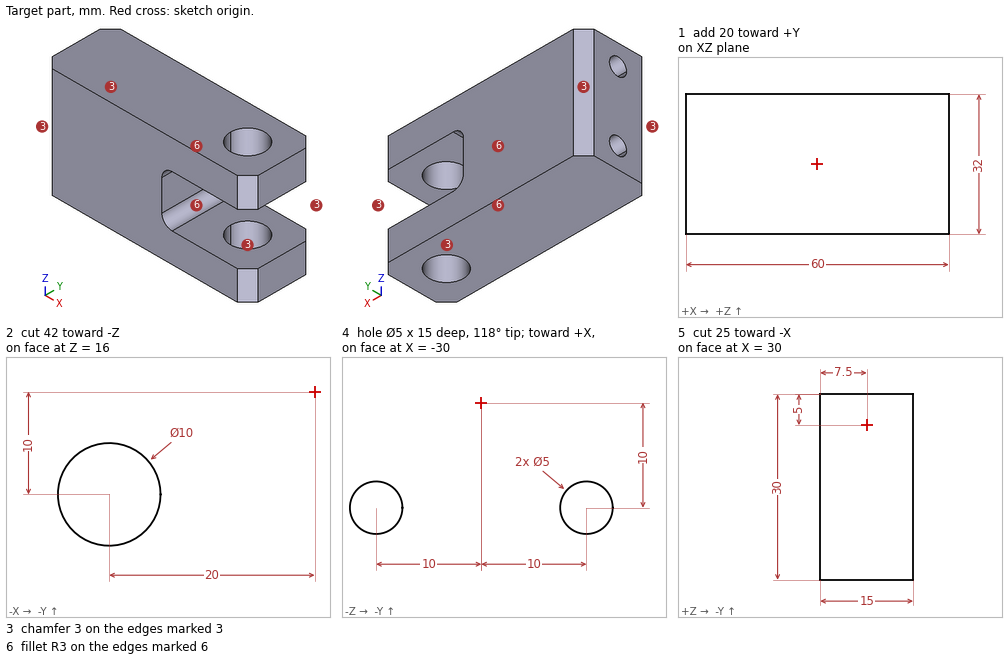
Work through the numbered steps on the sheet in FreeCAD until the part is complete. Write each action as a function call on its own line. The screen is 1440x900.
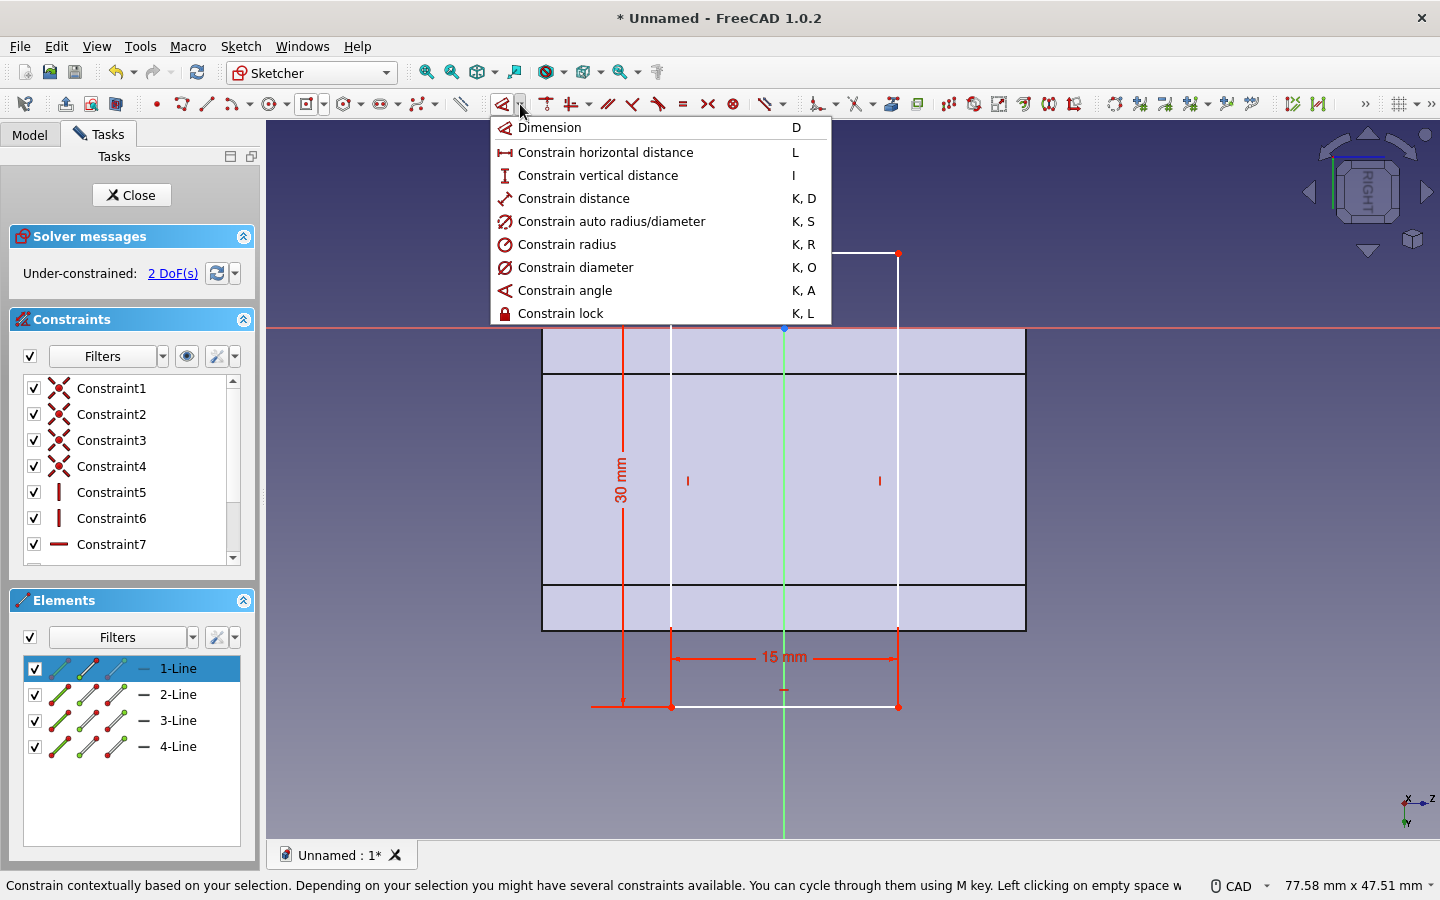
click(661, 176)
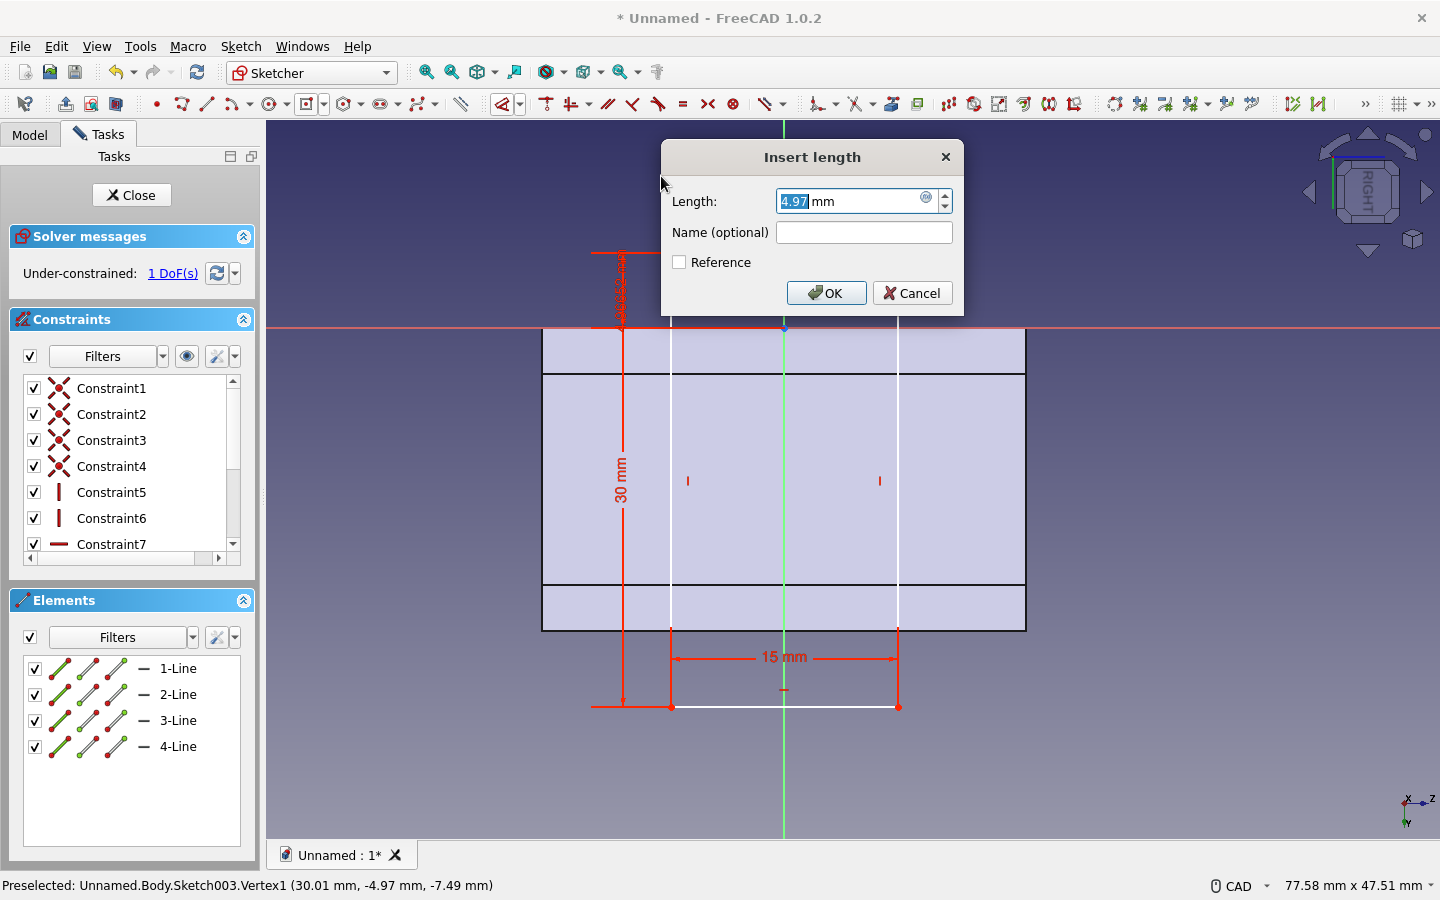
text(5)
key(Return)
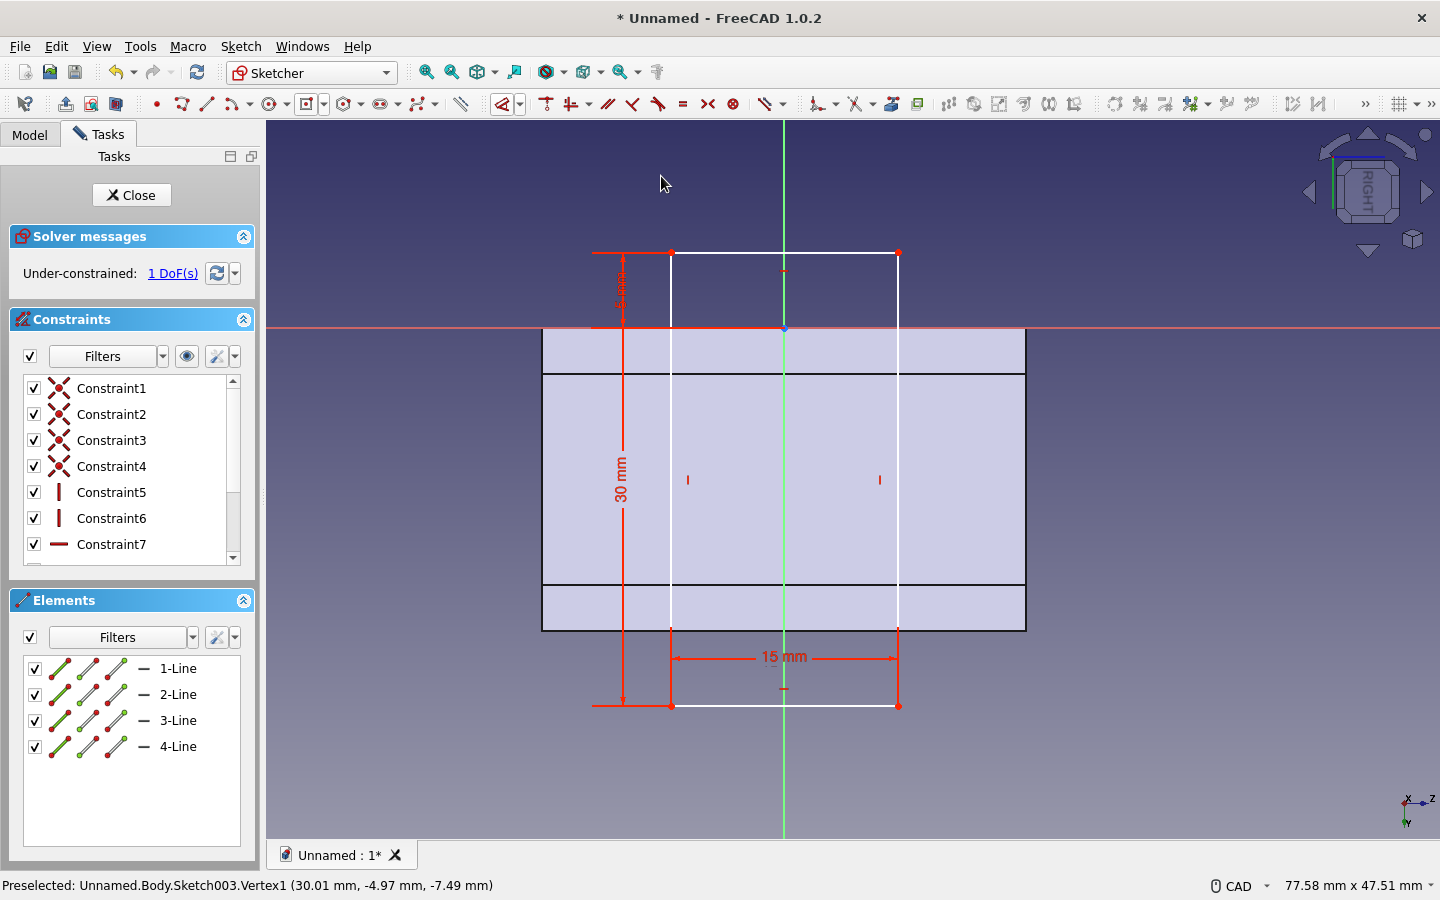
click(671, 253)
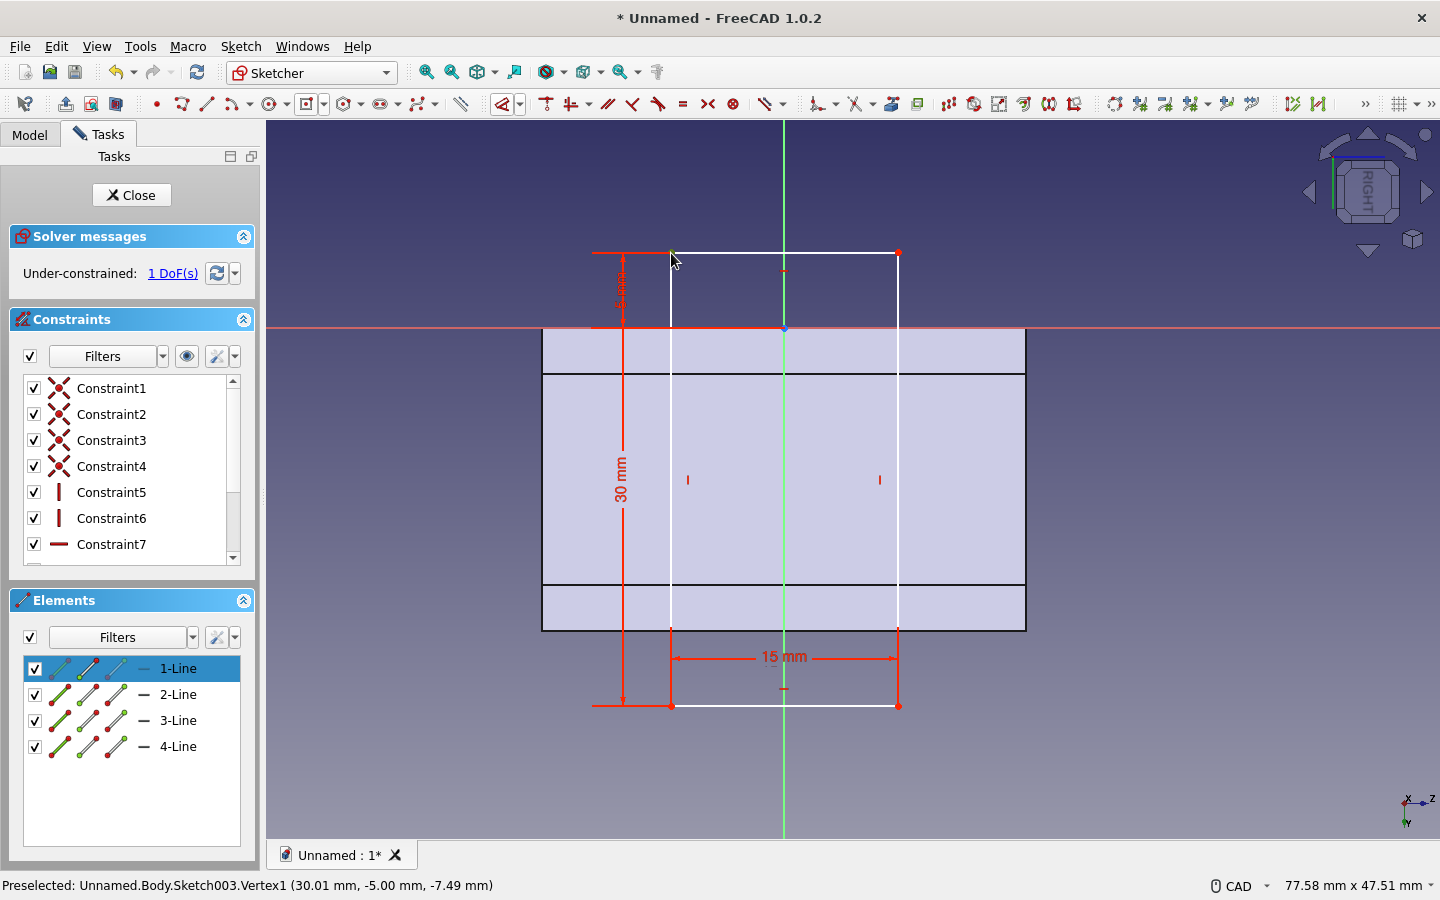
click(520, 104)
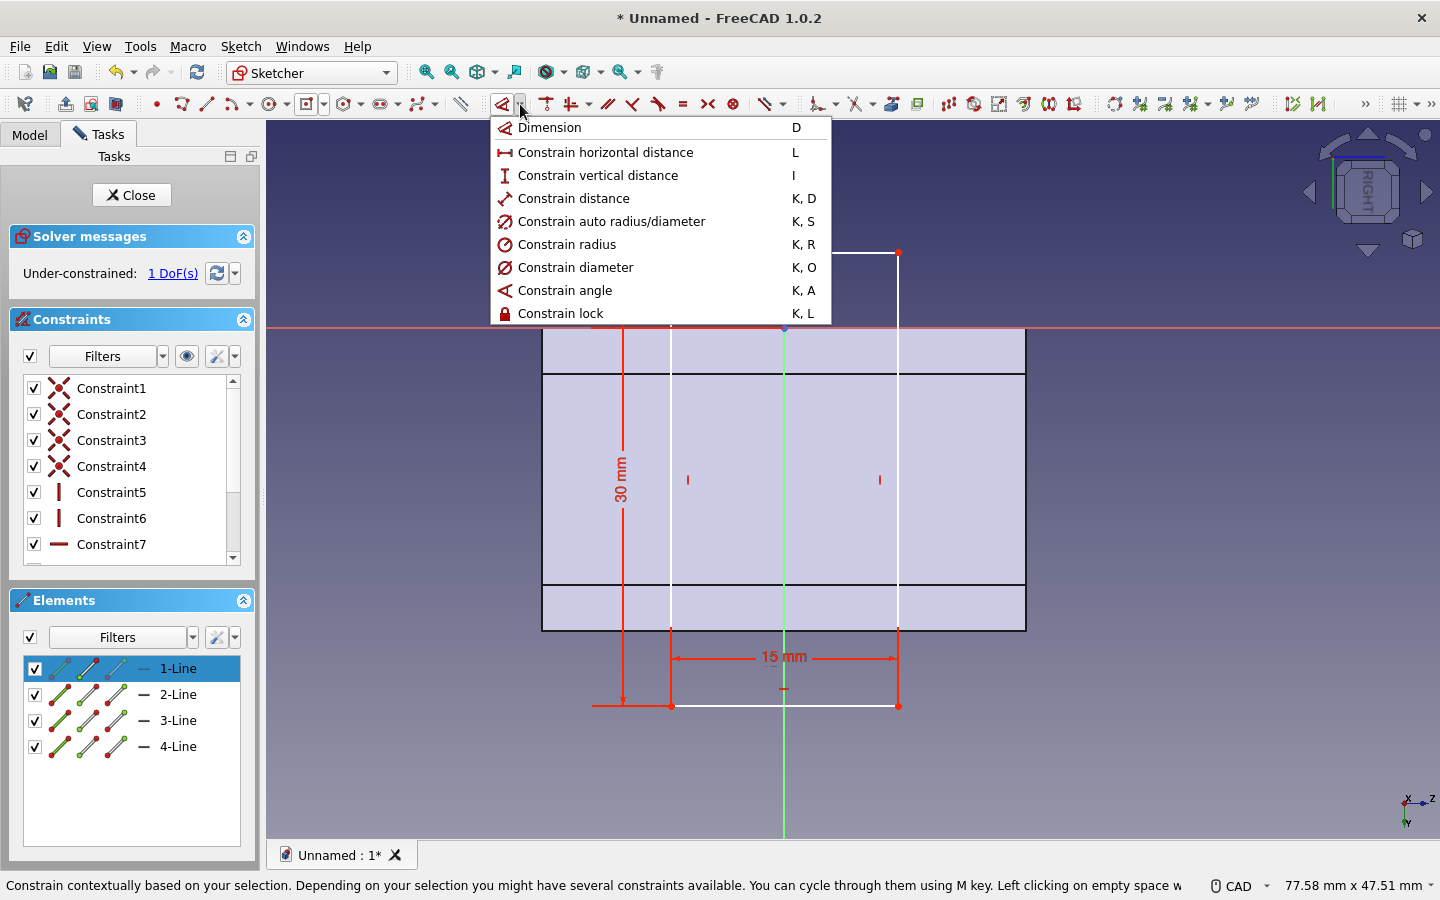
click(661, 152)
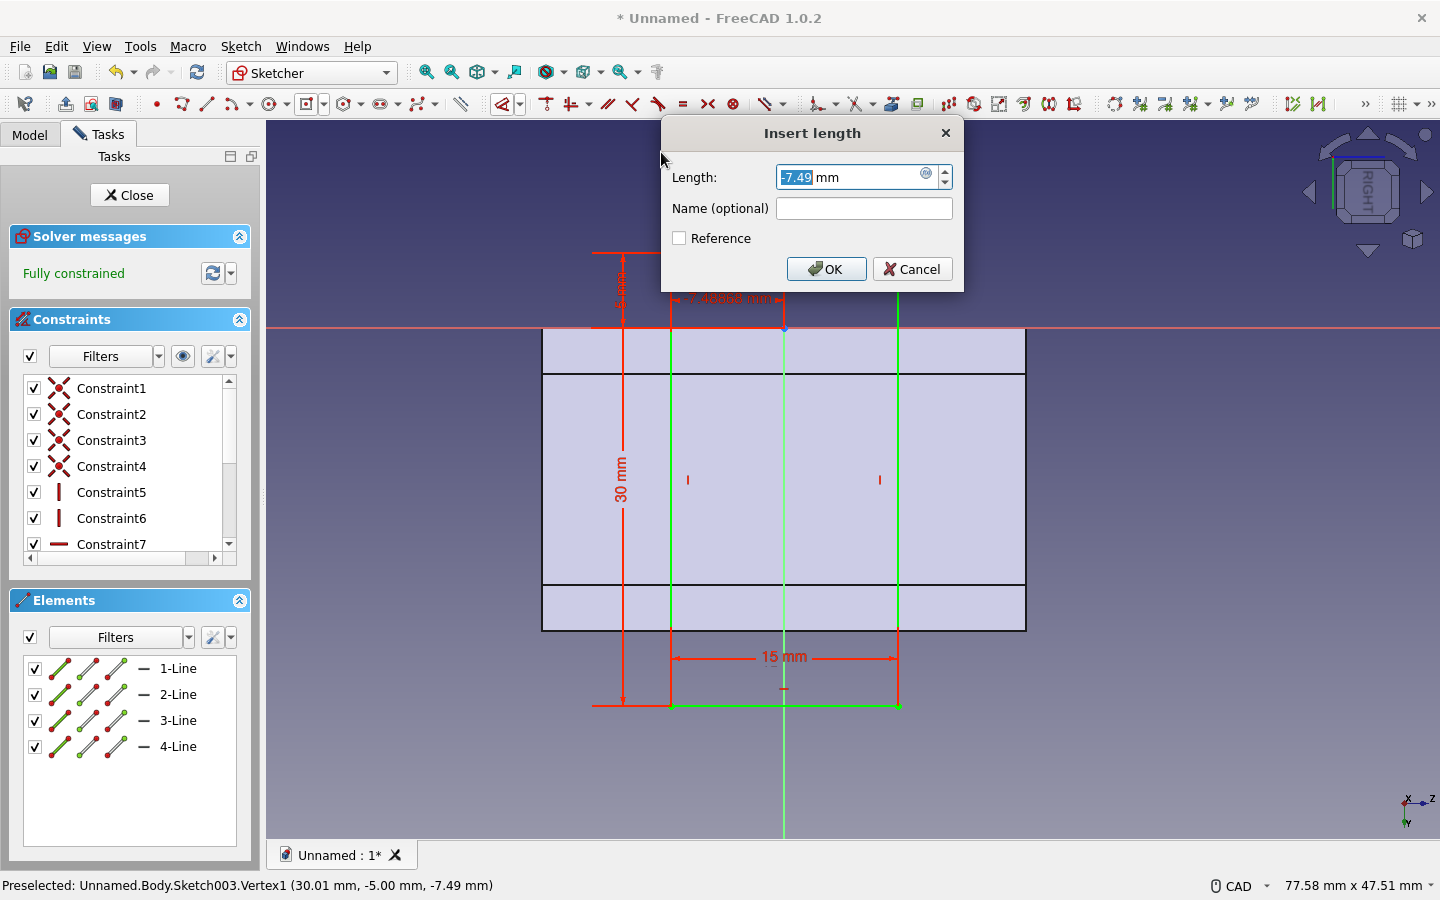
text(-7.5)
key(Return)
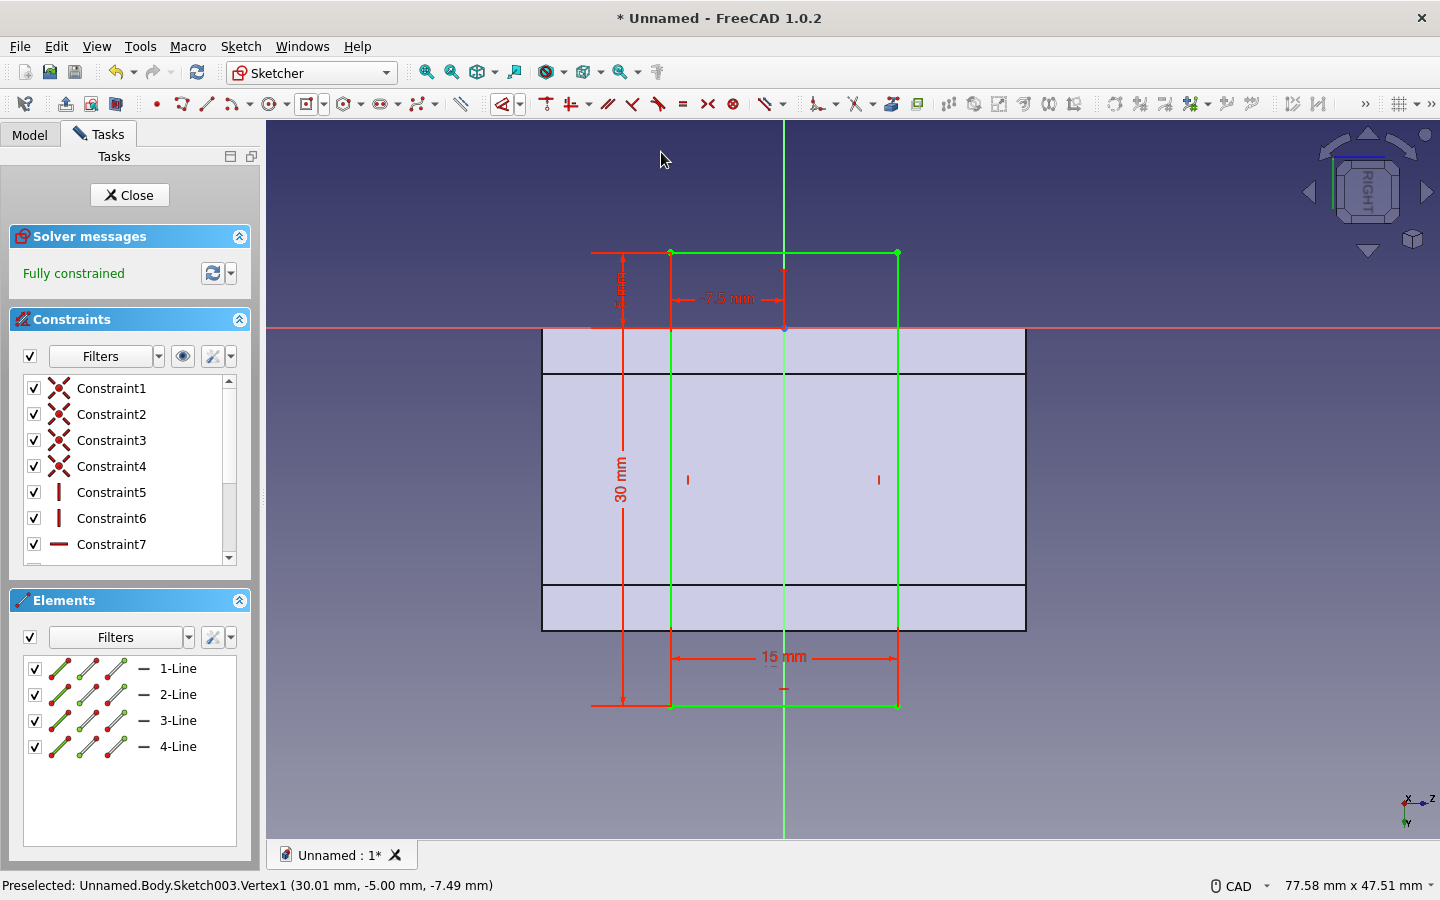
click(130, 195)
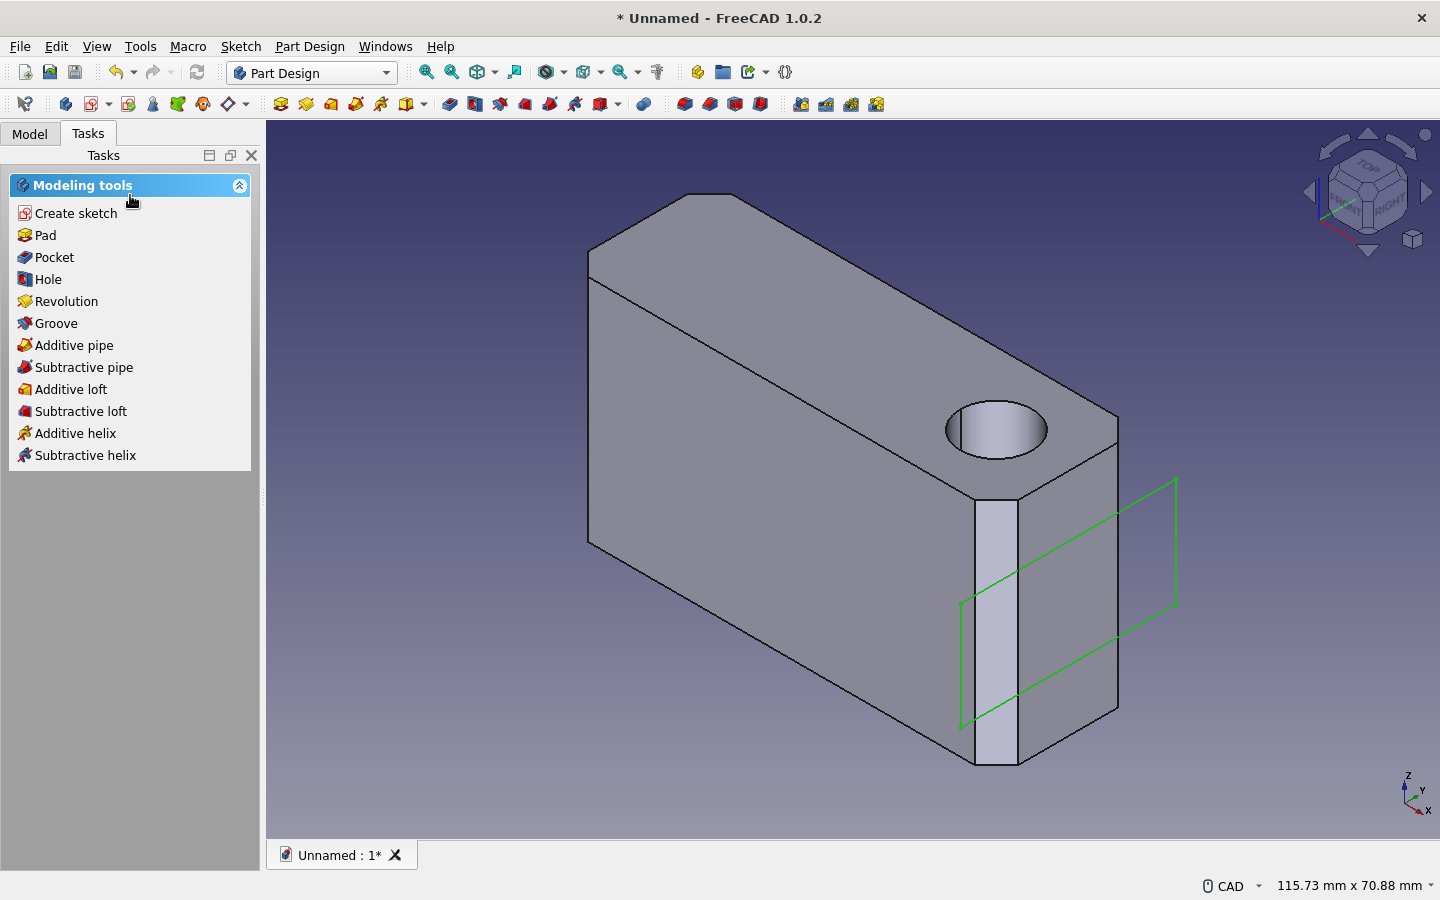
click(450, 104)